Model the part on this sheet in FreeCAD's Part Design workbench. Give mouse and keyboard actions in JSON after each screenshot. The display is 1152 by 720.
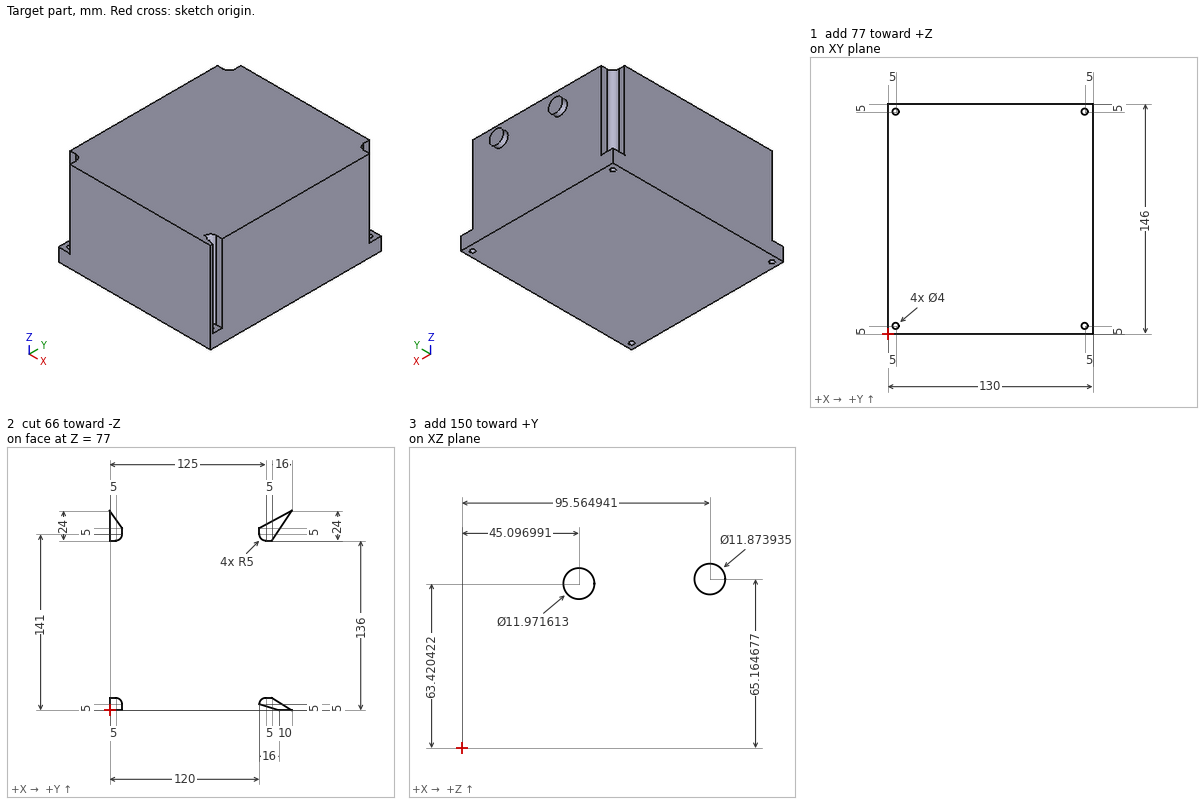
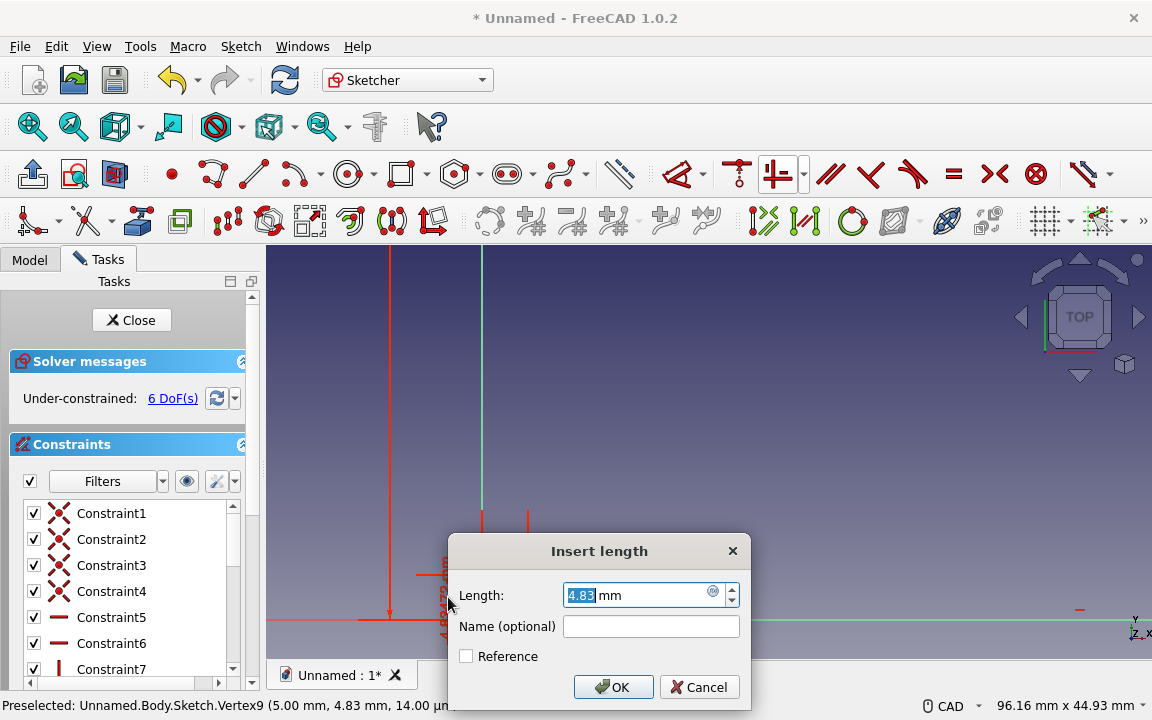
{"action": "type", "text": "5"}
{"action": "key", "text": "Return"}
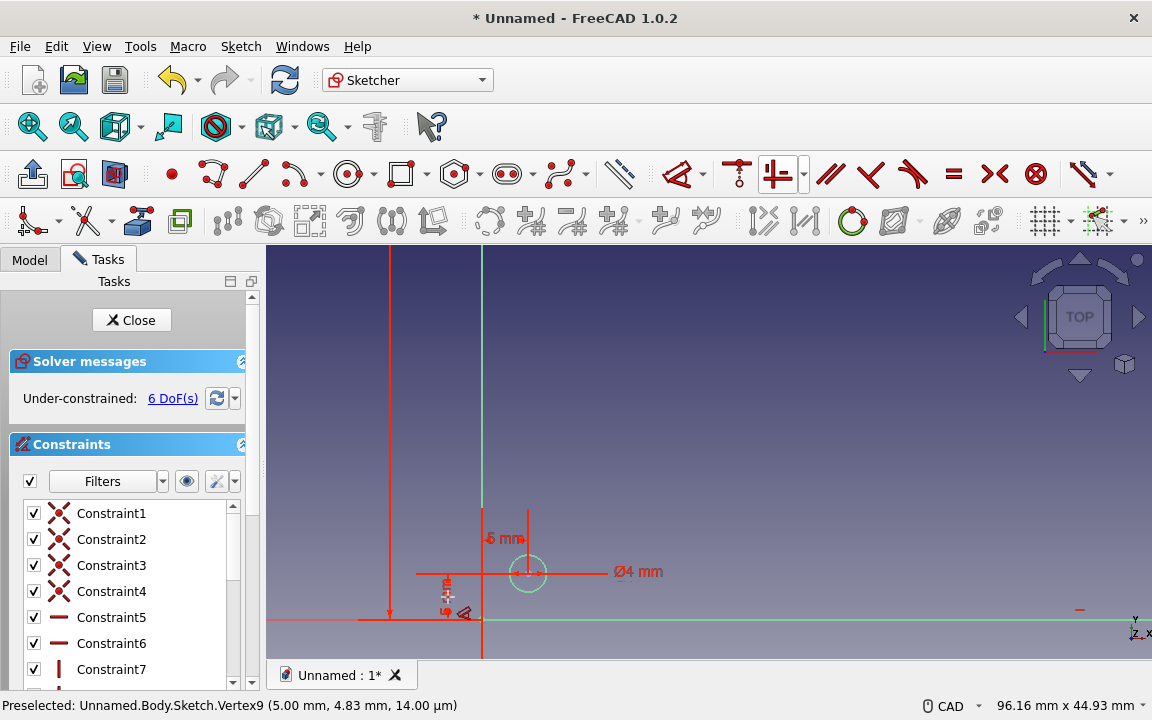
{"action": "scroll", "coordinate": [529, 580], "scroll_direction": "down", "scroll_amount": 8}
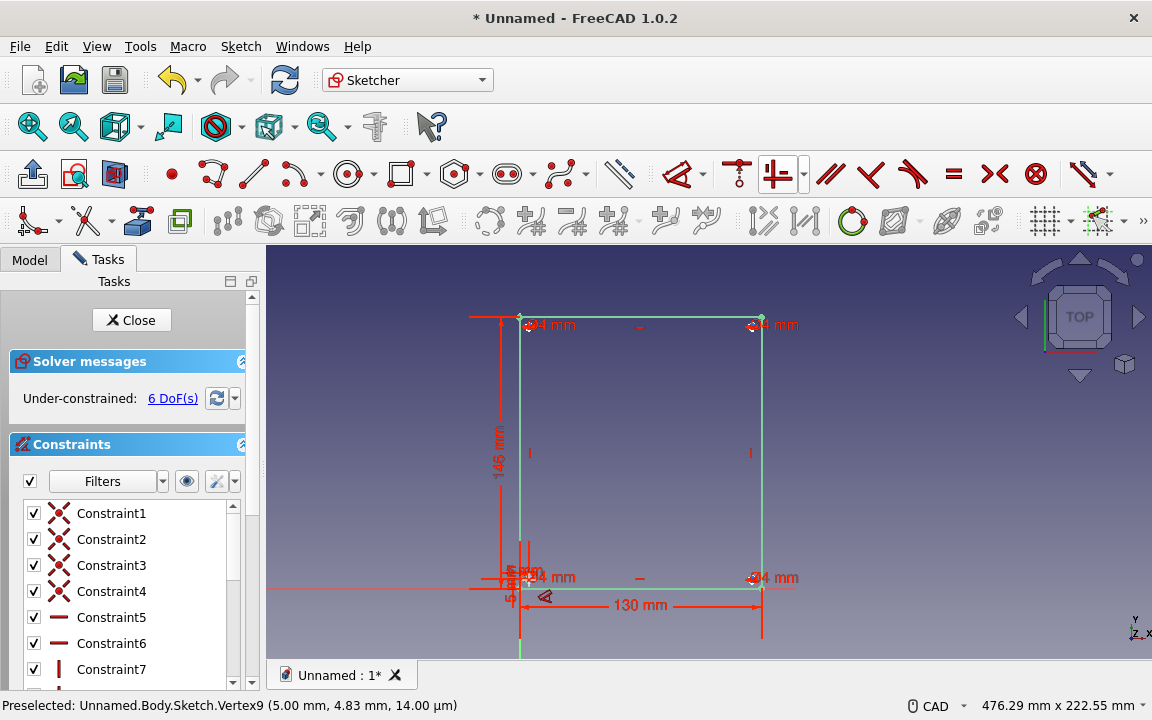
{"action": "scroll", "coordinate": [752, 580], "scroll_direction": "up", "scroll_amount": 8}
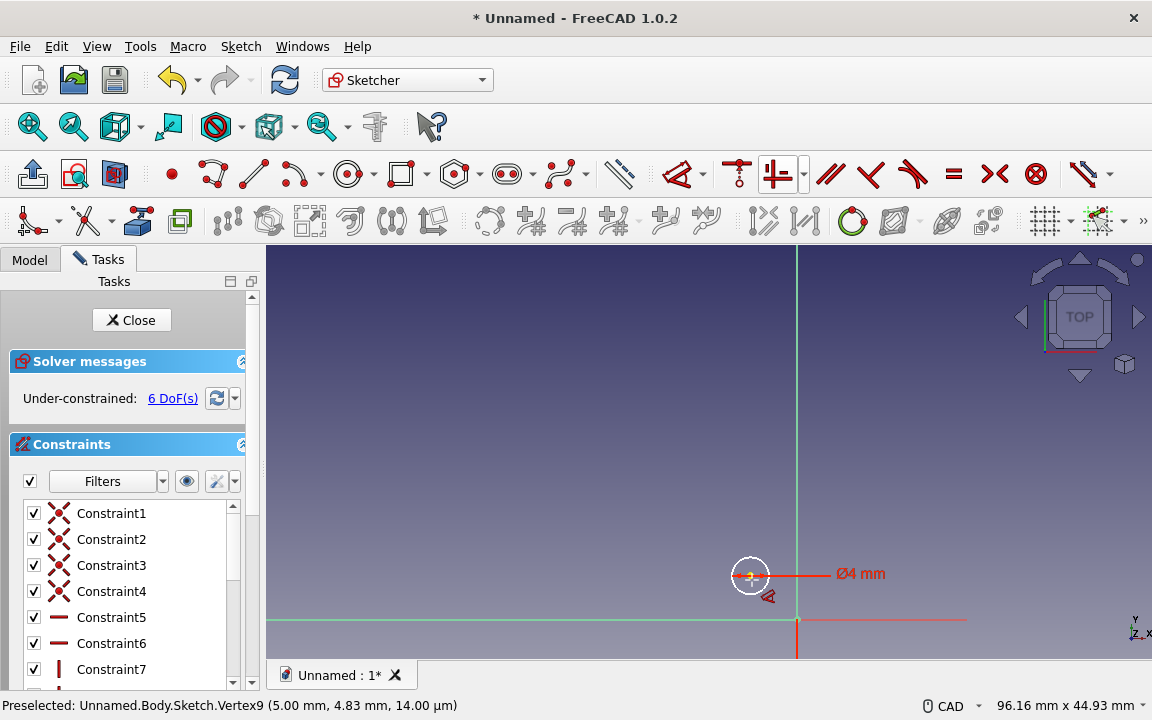
{"action": "left_click", "coordinate": [750, 576]}
{"action": "left_click", "coordinate": [832, 598]}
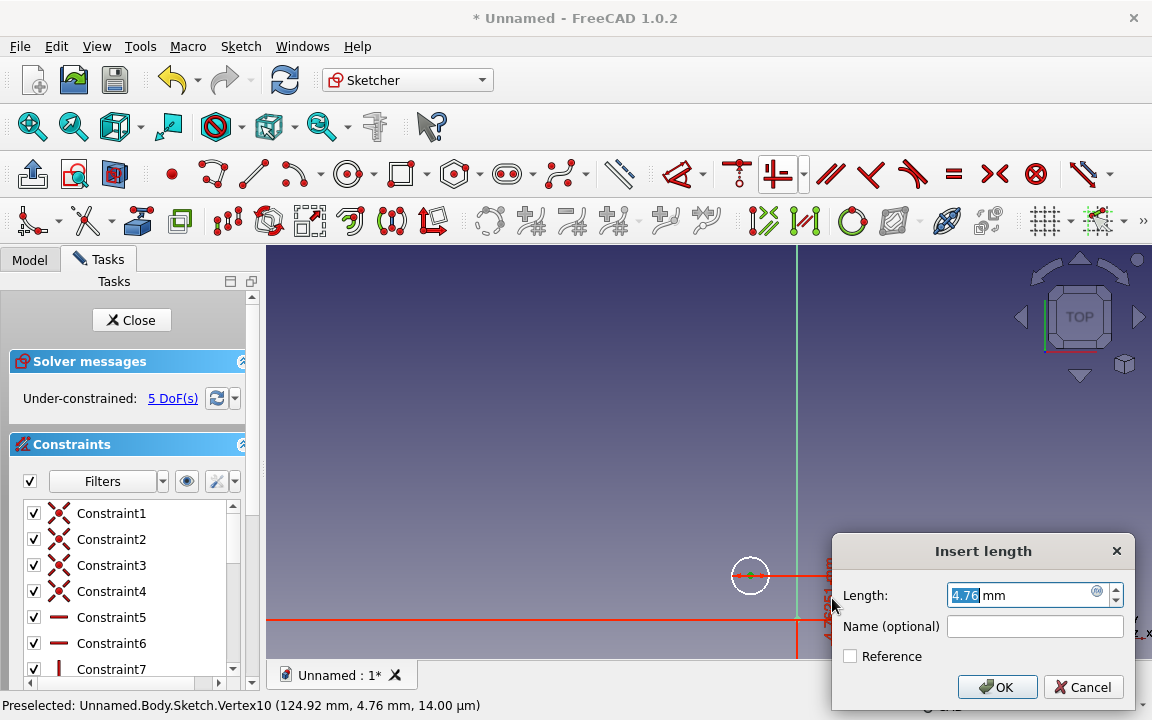
{"action": "type", "text": "5"}
{"action": "key", "text": "Return"}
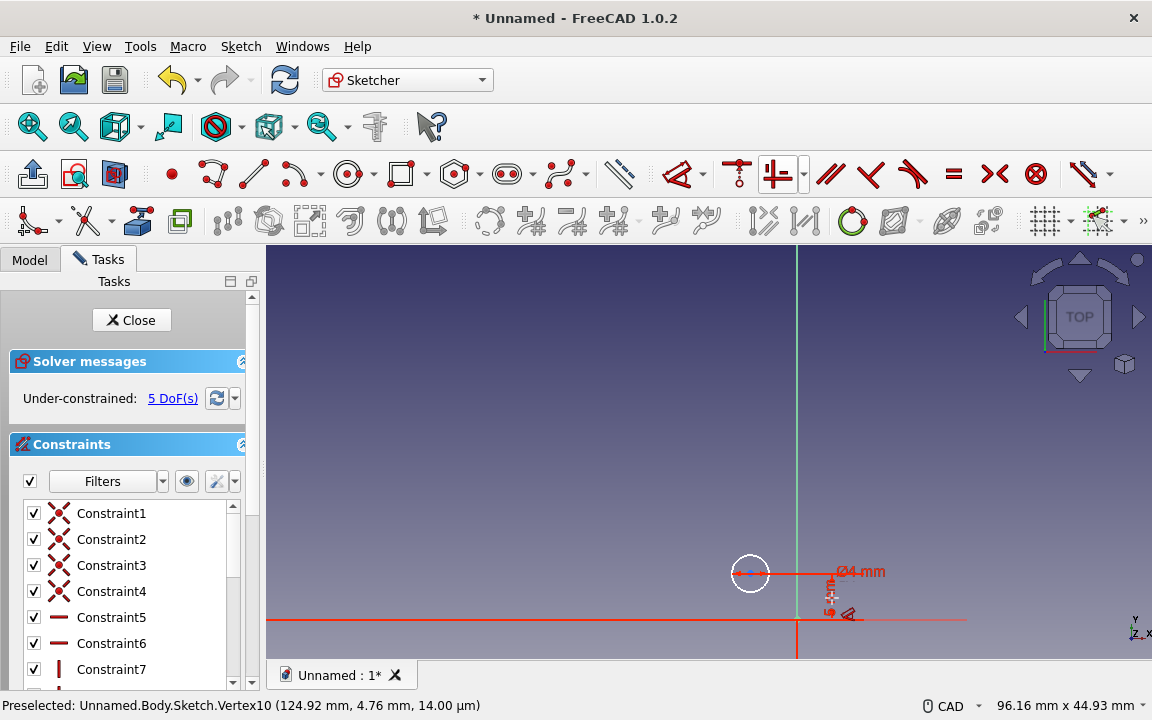
{"action": "scroll", "coordinate": [752, 580], "scroll_direction": "down", "scroll_amount": 8}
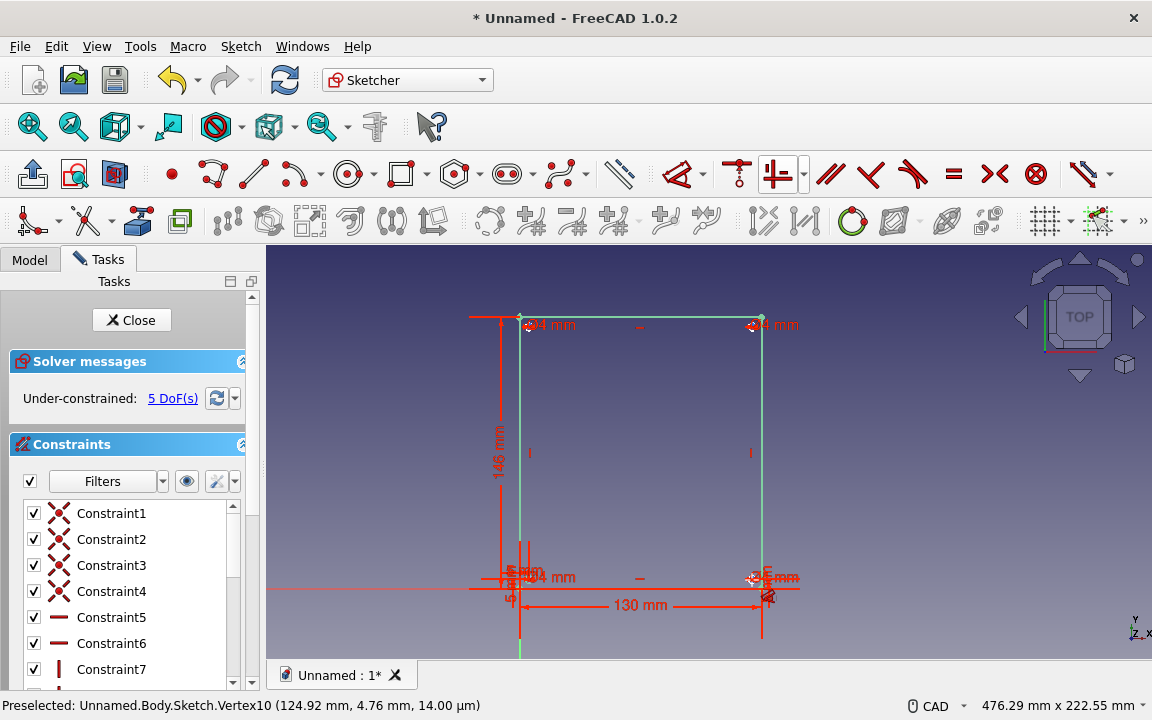
{"action": "scroll", "coordinate": [529, 327], "scroll_direction": "up", "scroll_amount": 8}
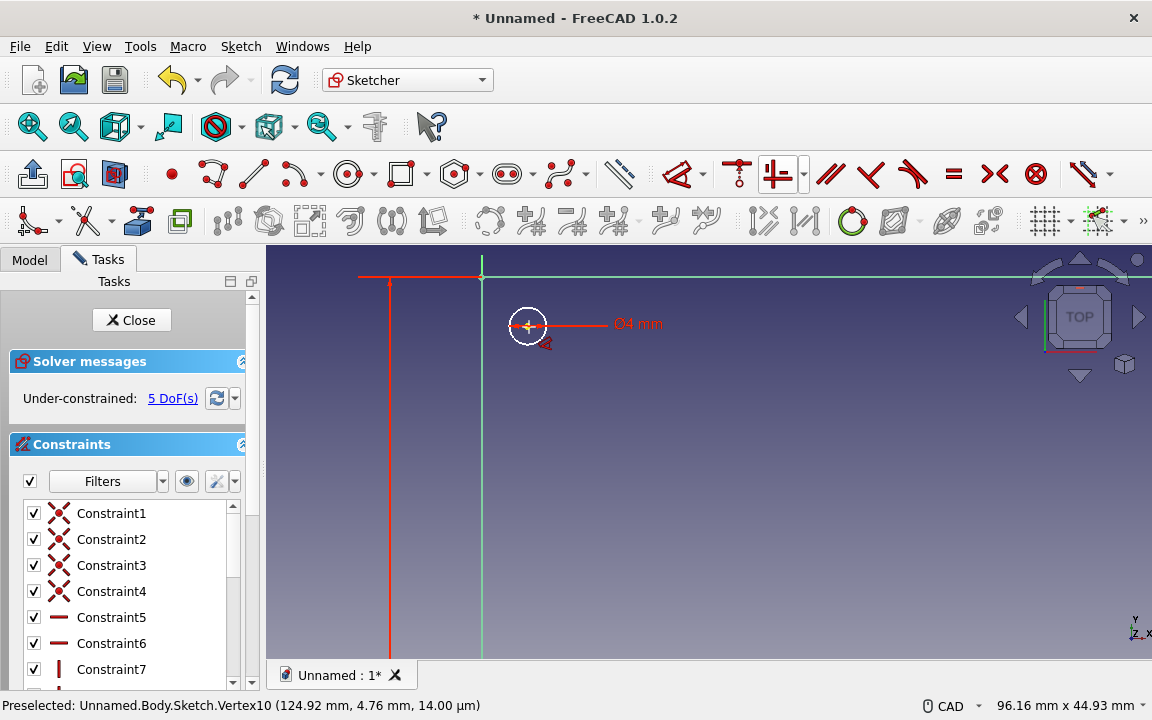
{"action": "left_click", "coordinate": [528, 326]}
{"action": "left_click", "coordinate": [505, 292]}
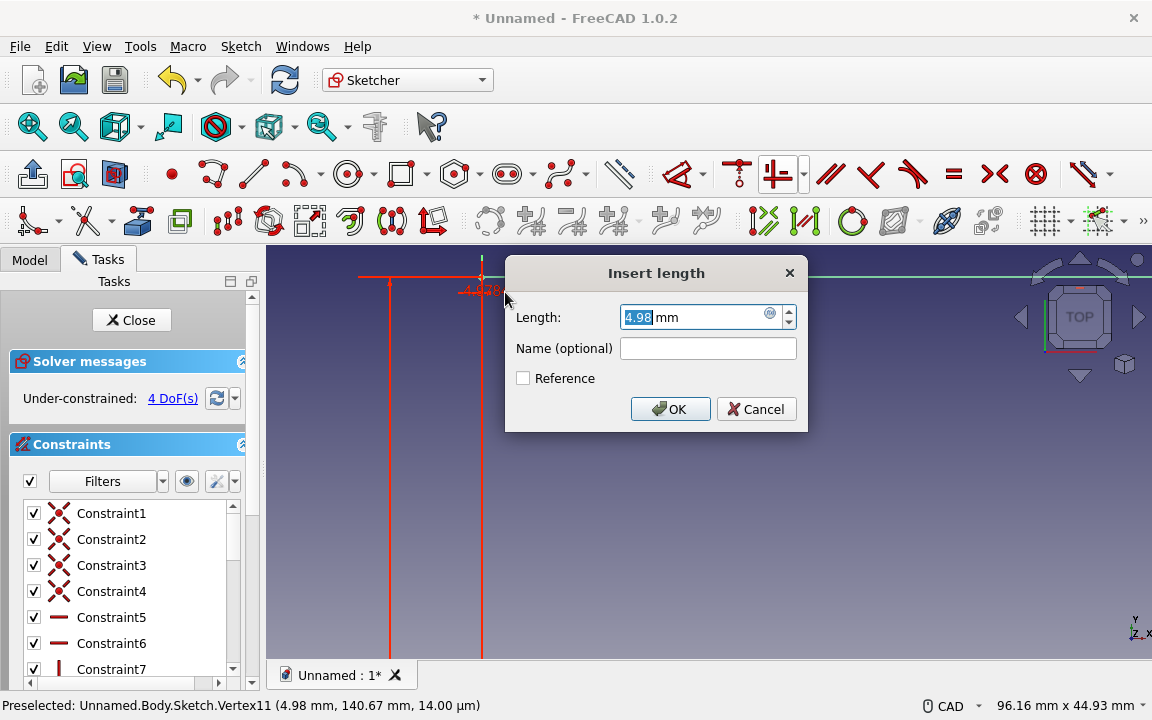
{"action": "type", "text": "5"}
{"action": "key", "text": "Return"}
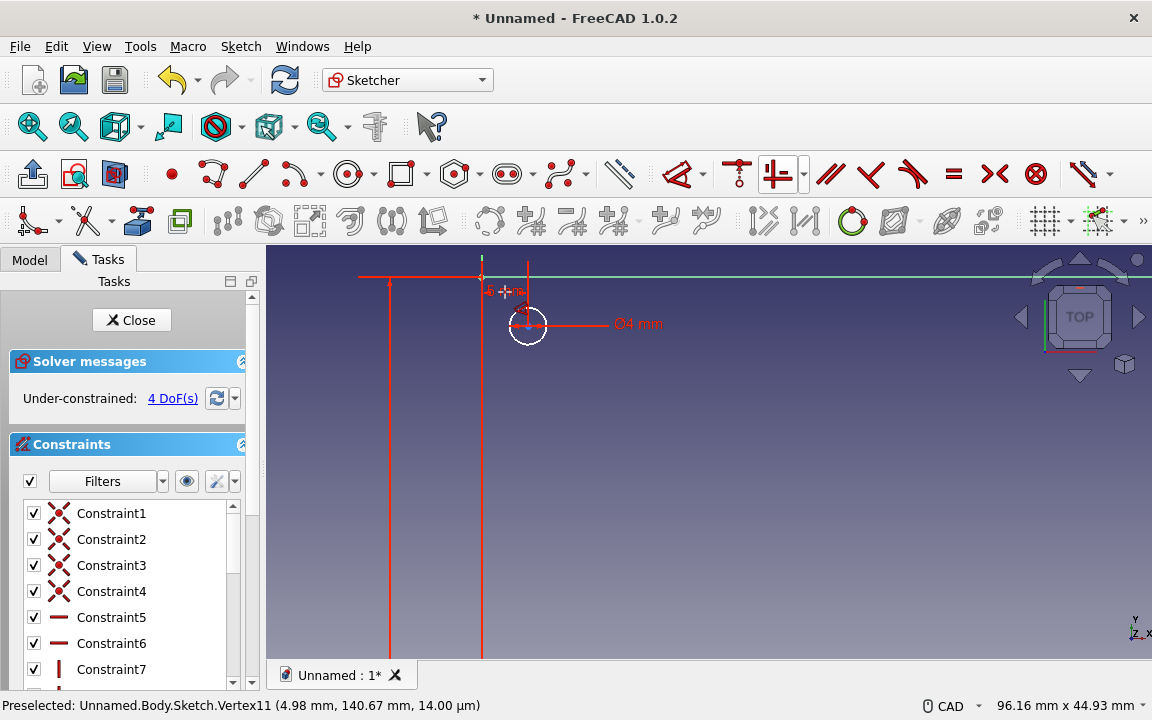
{"action": "scroll", "coordinate": [529, 326], "scroll_direction": "down", "scroll_amount": 8}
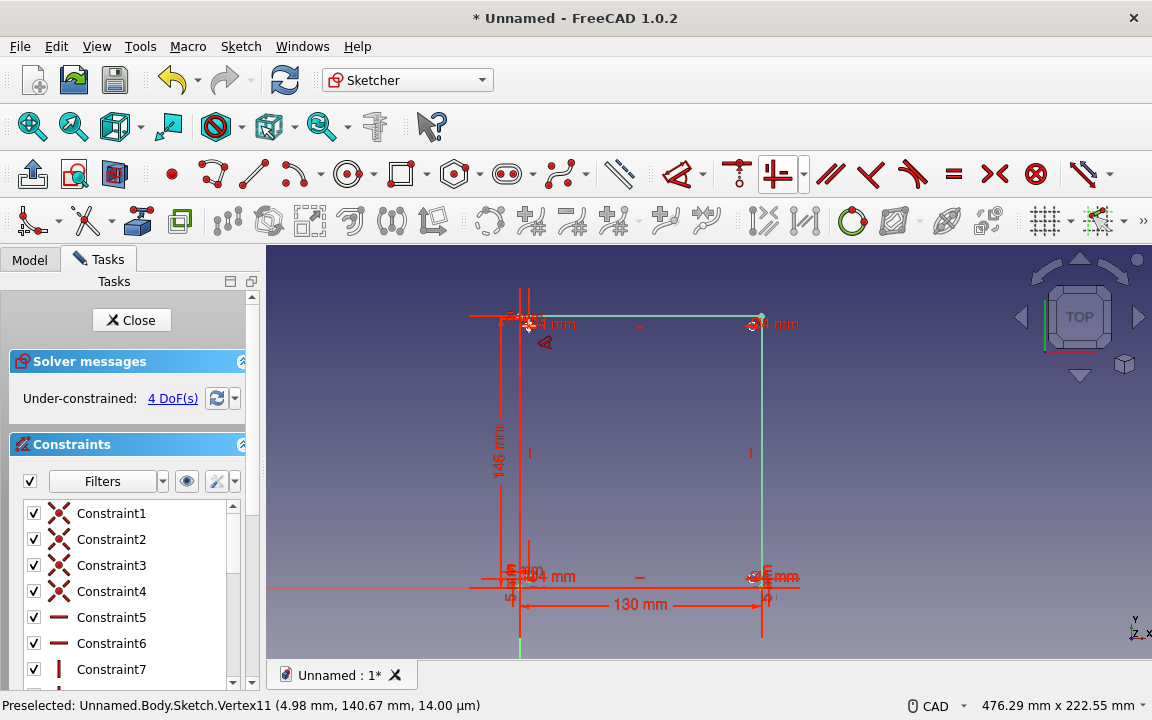
{"action": "scroll", "coordinate": [762, 588], "scroll_direction": "up", "scroll_amount": 8}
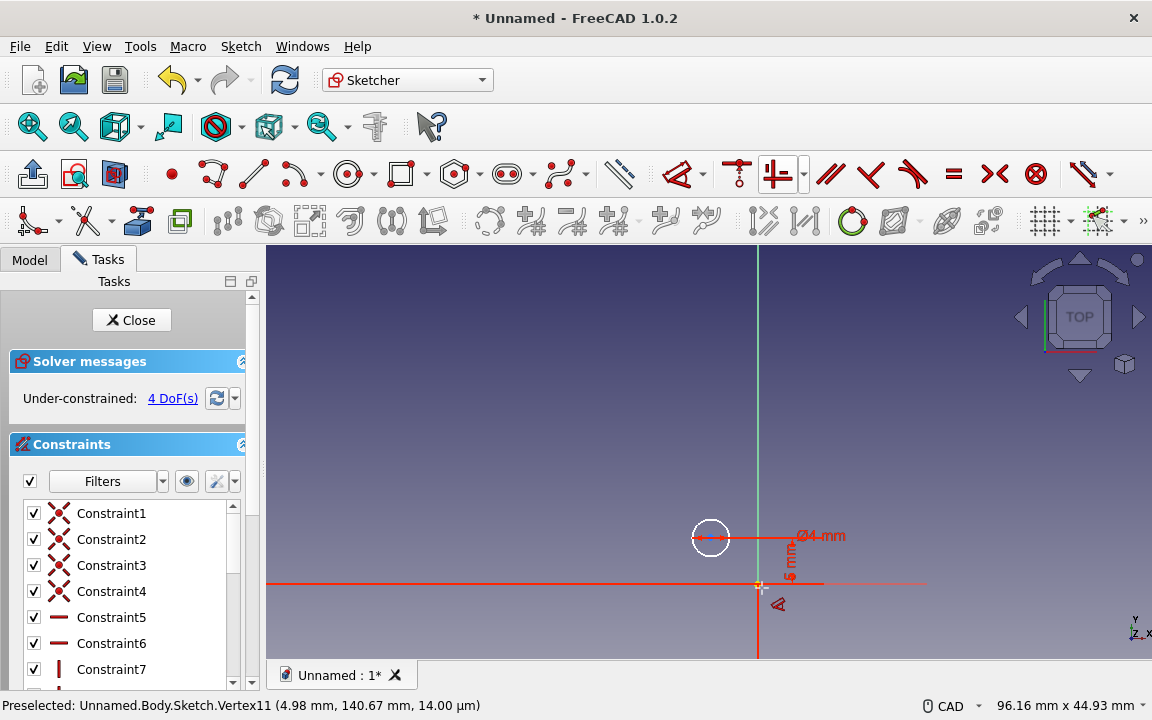
{"action": "left_click", "coordinate": [758, 584]}